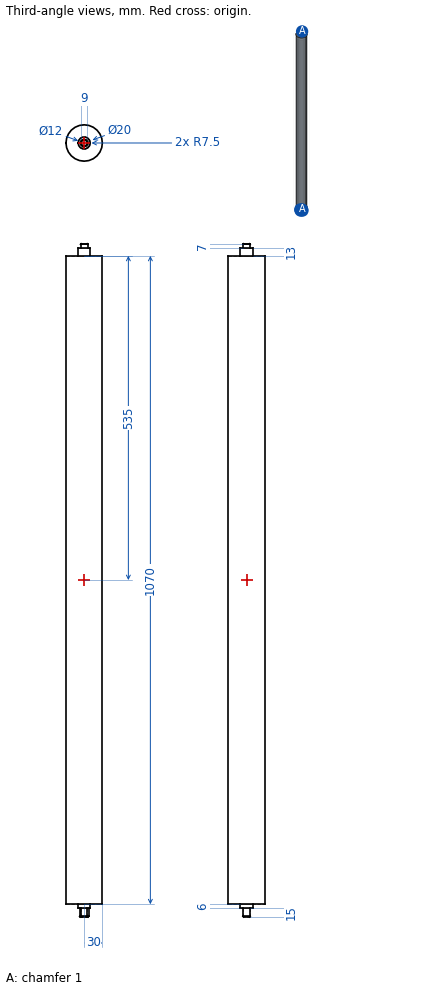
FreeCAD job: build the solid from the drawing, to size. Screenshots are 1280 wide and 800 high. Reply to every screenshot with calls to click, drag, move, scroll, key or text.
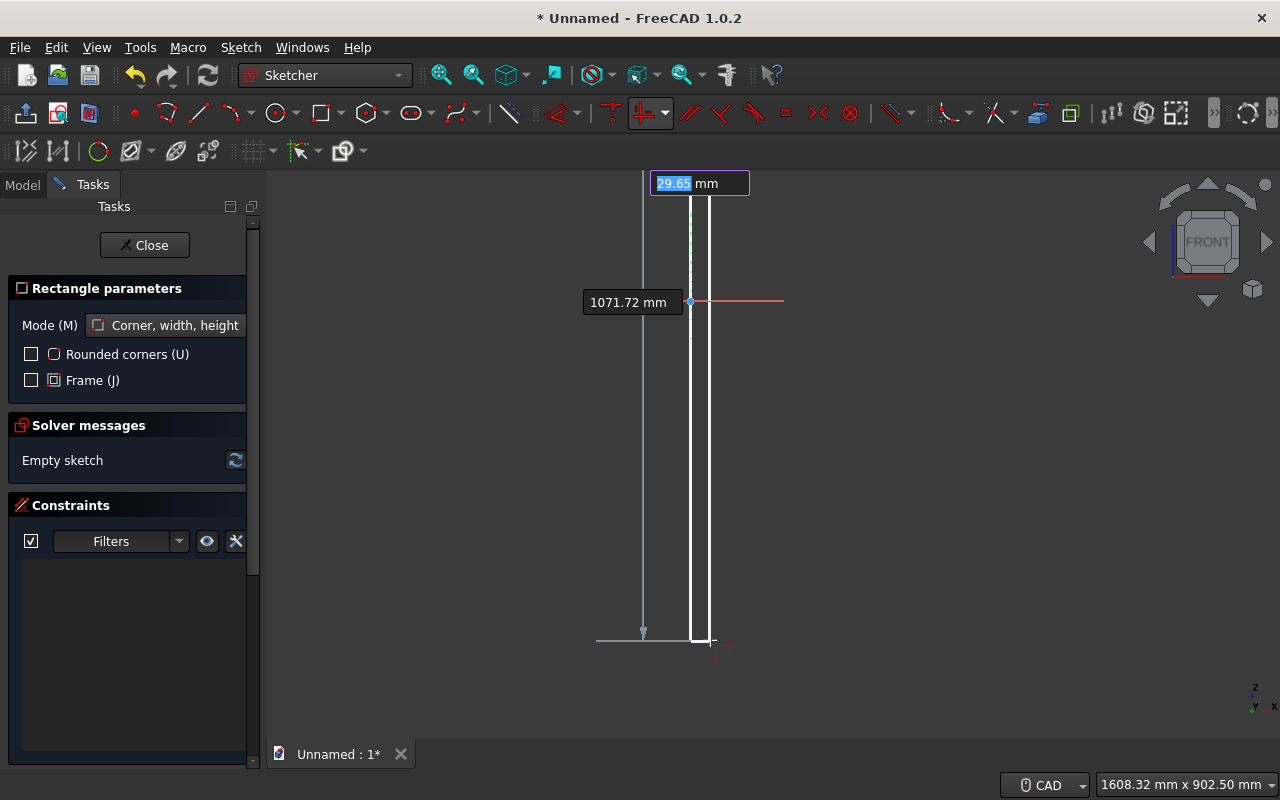
click(710, 639)
key(Escape)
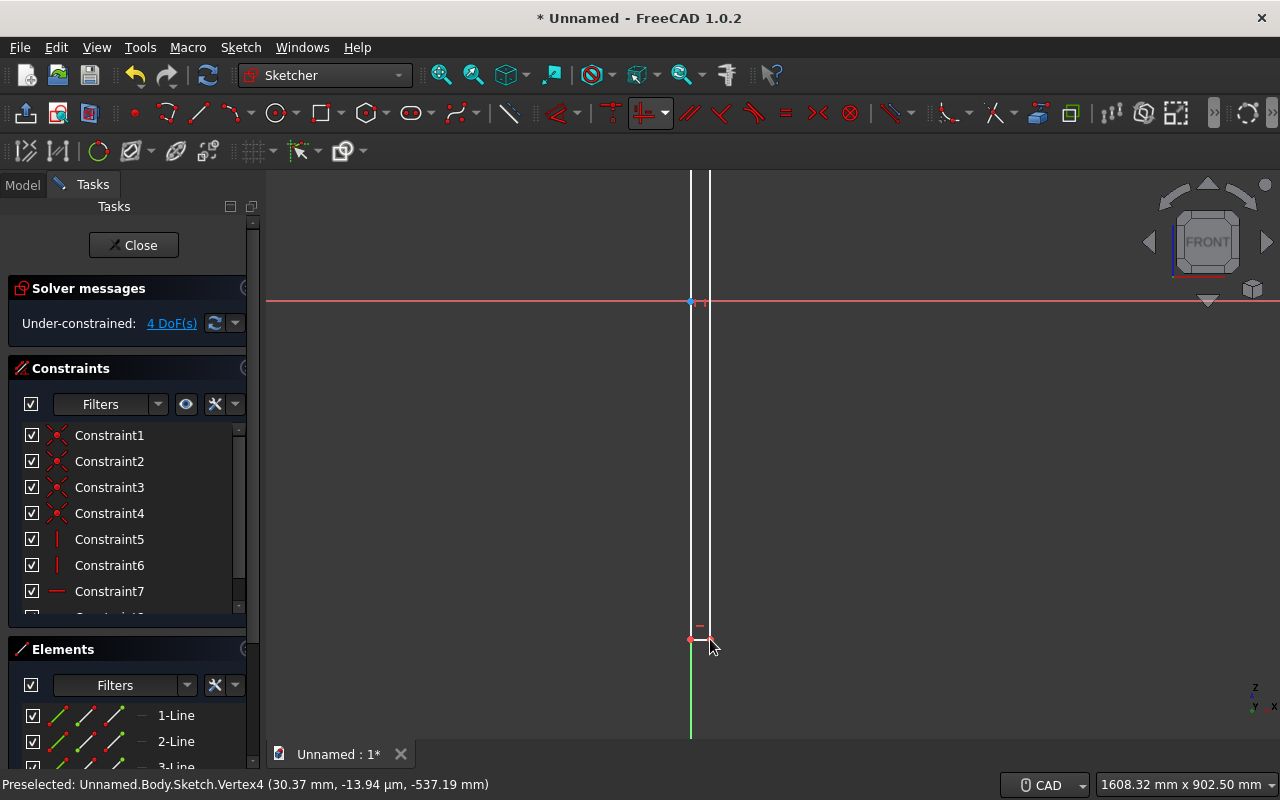
scroll(710, 641, down, 3)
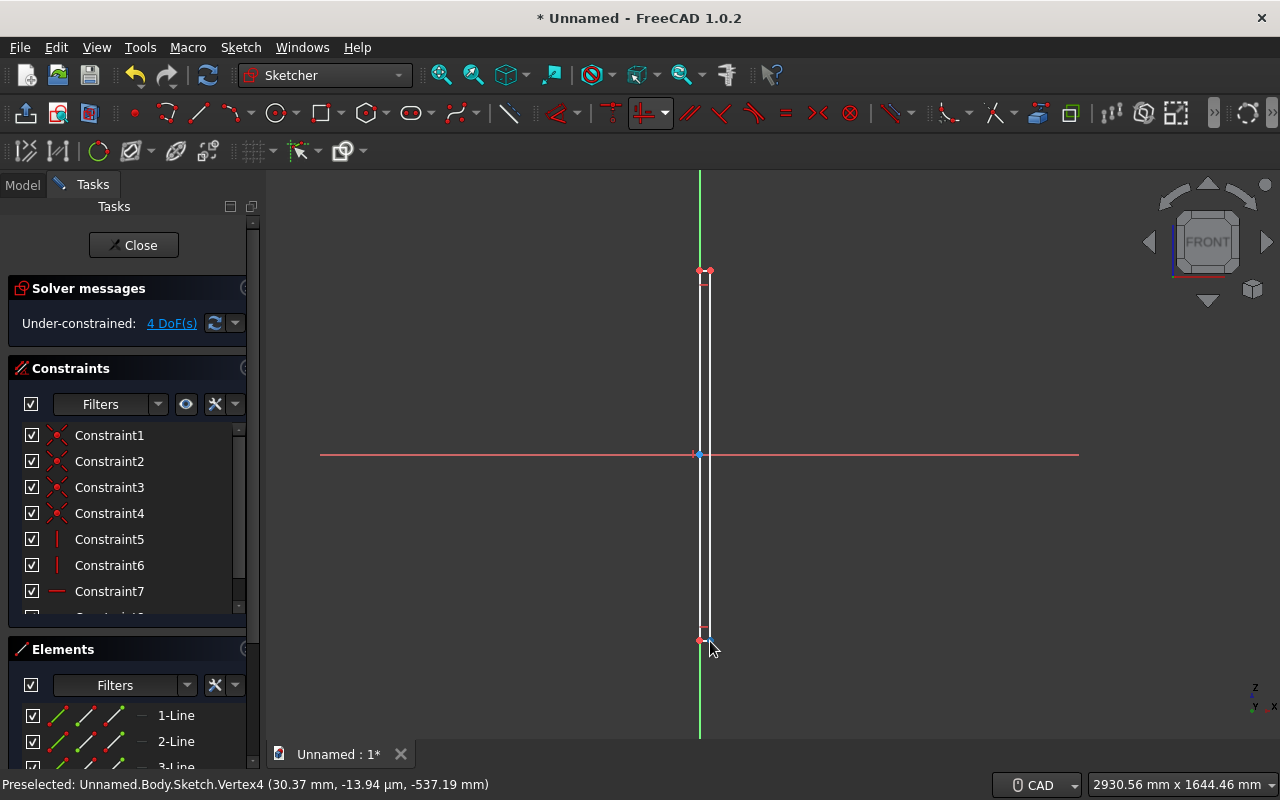
click(700, 271)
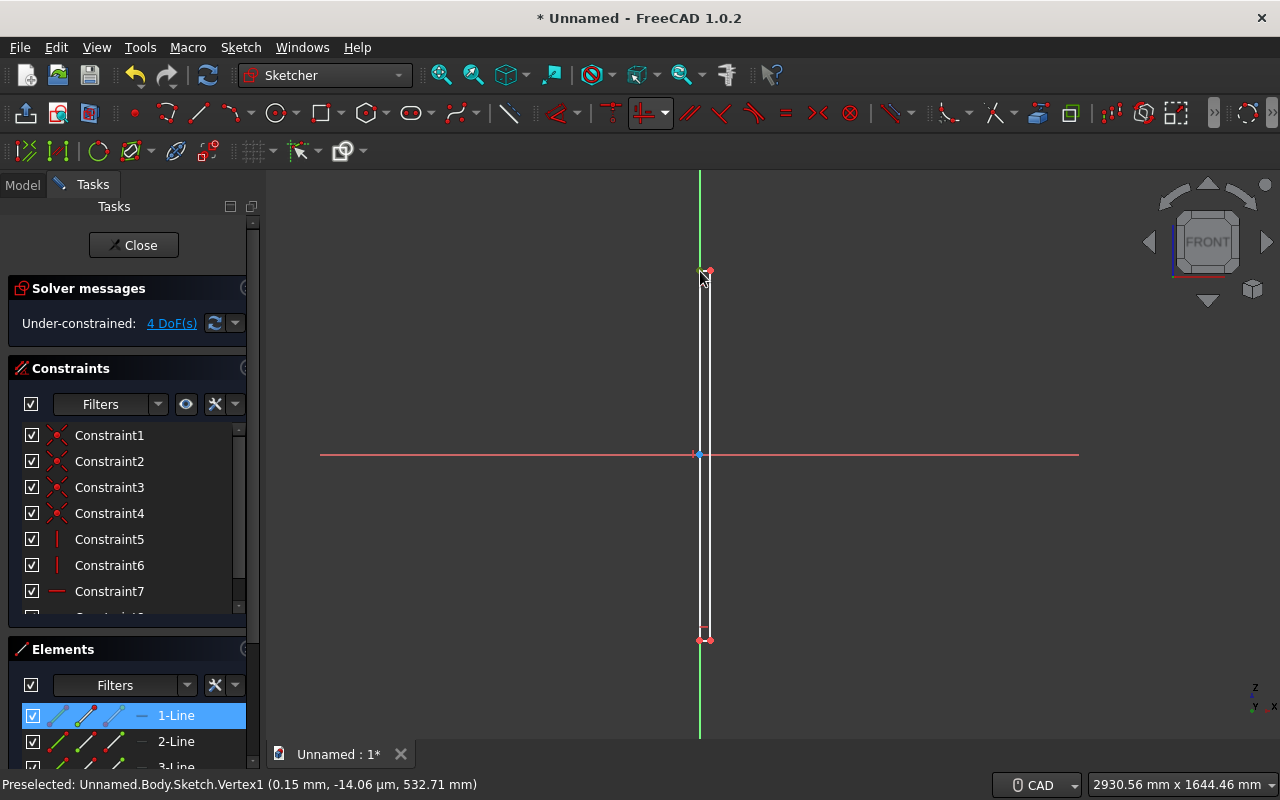
click(700, 674)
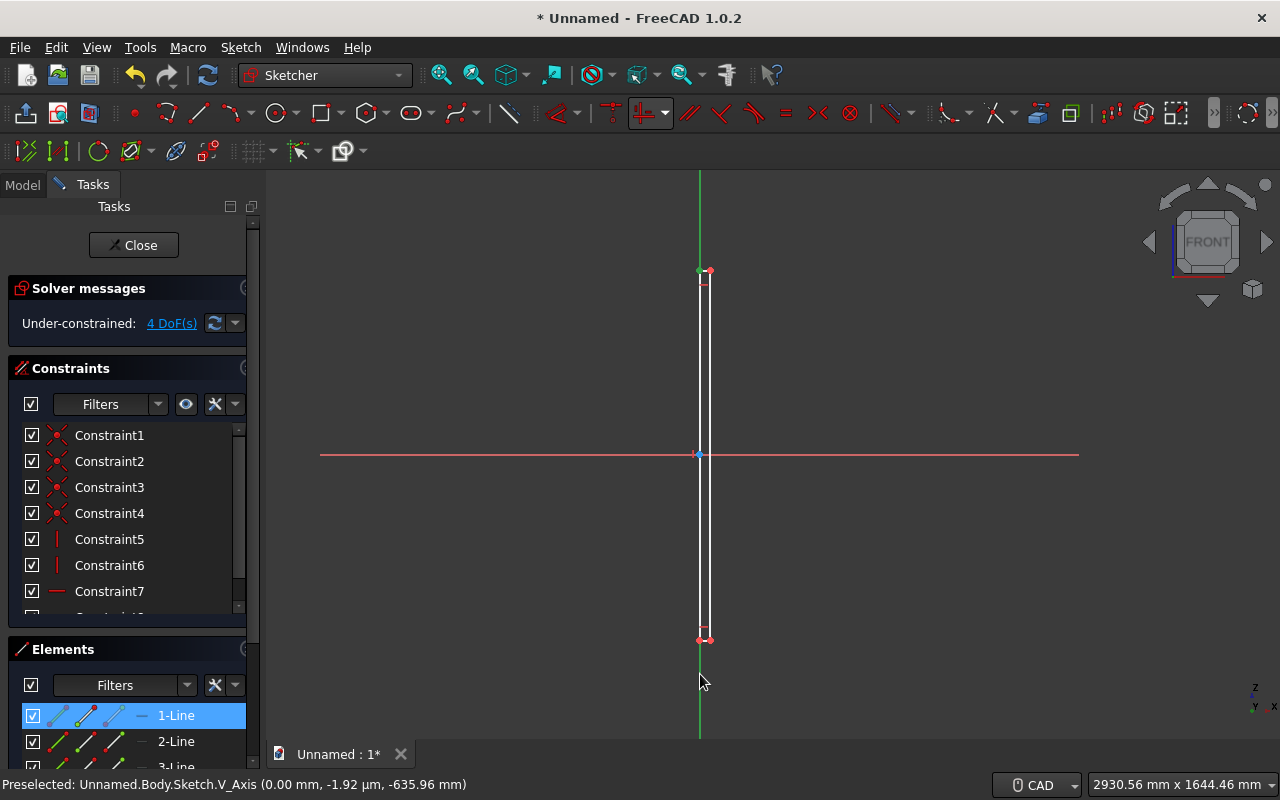
key(c)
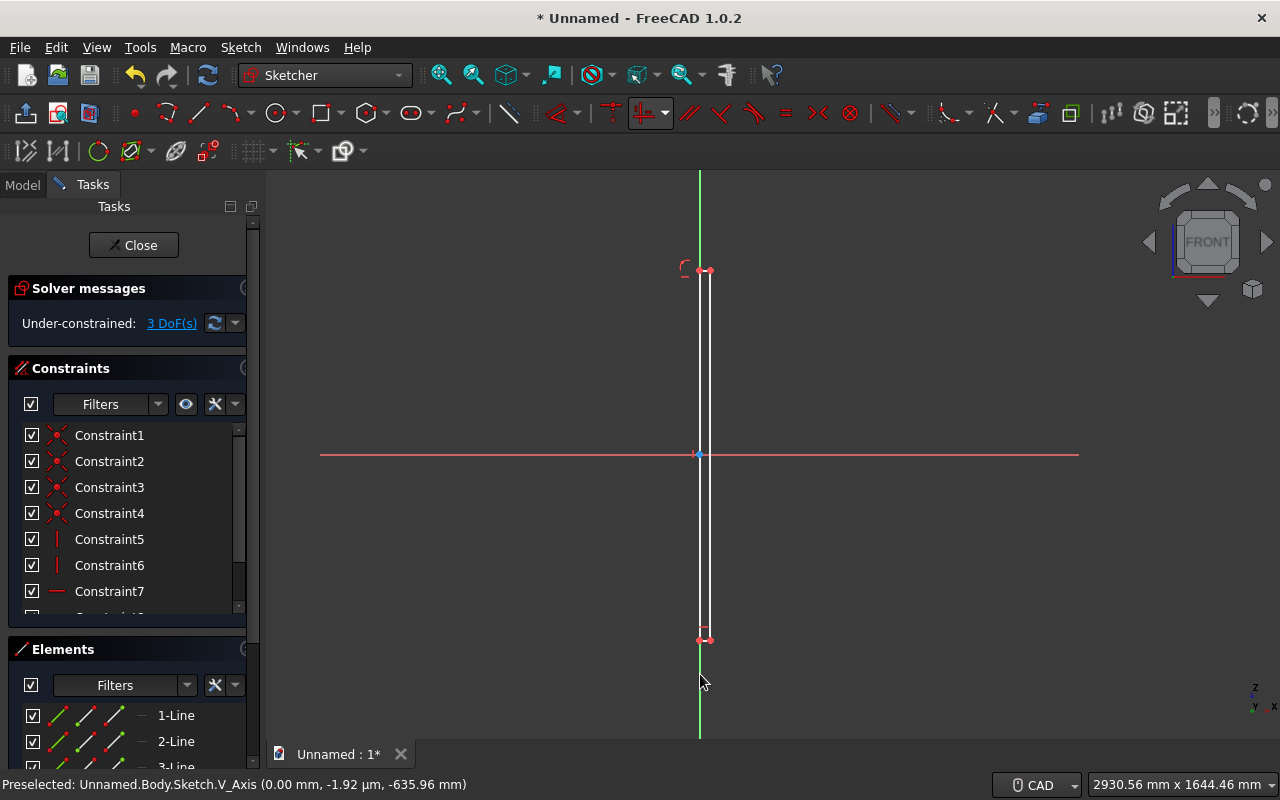
scroll(705, 641, up, 7)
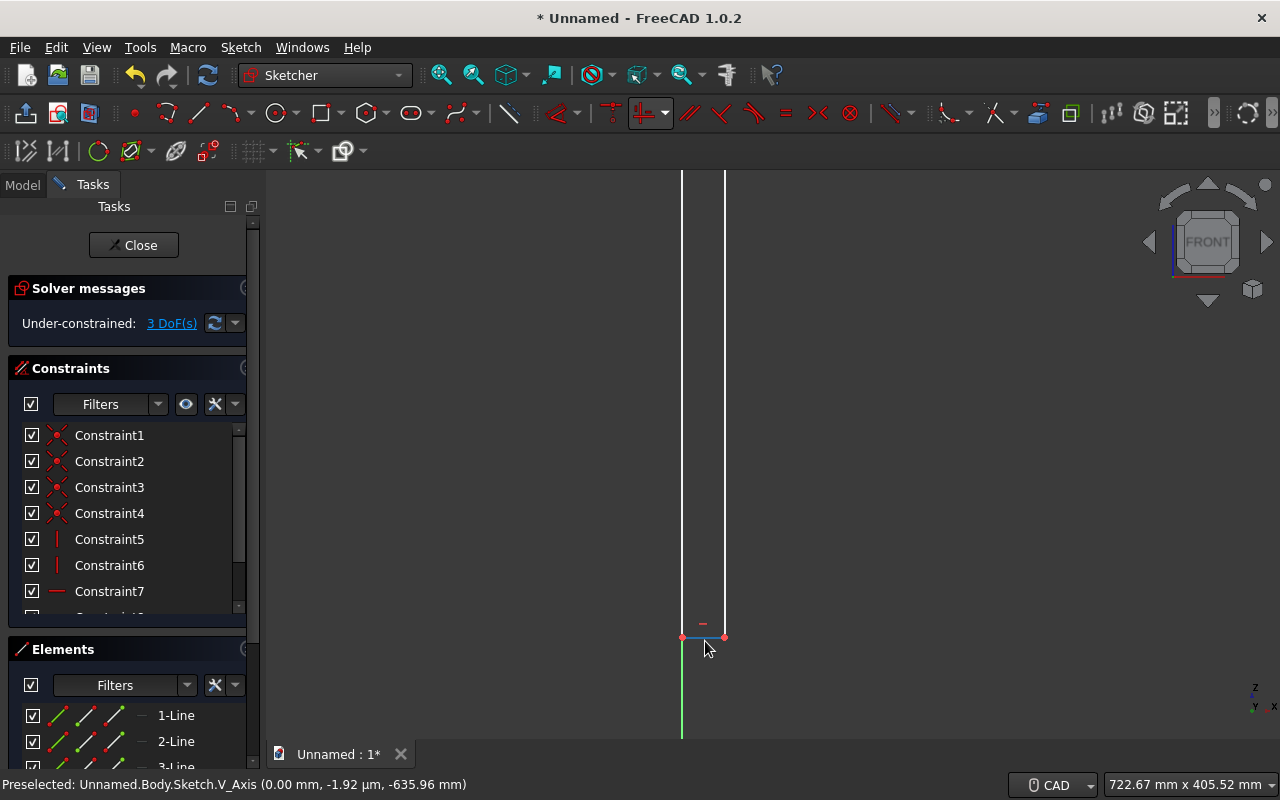
click(703, 638)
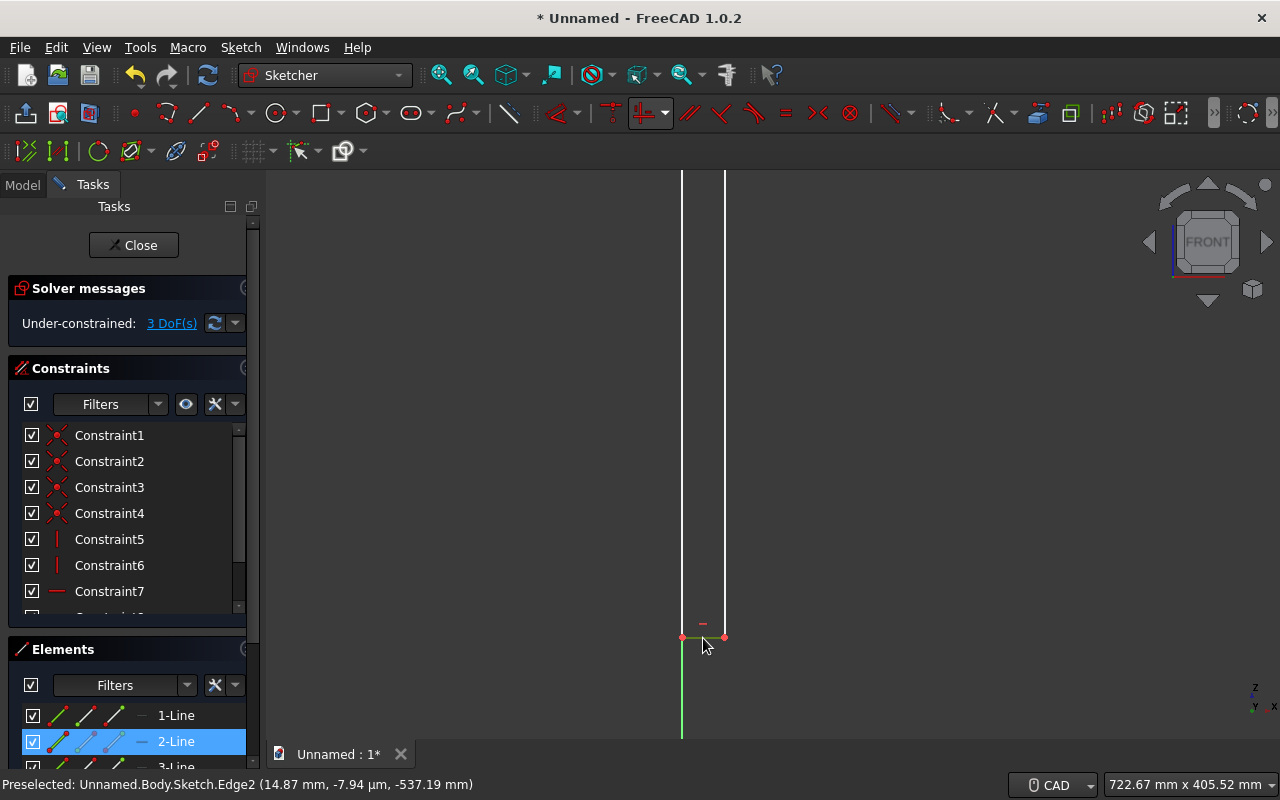
key(l)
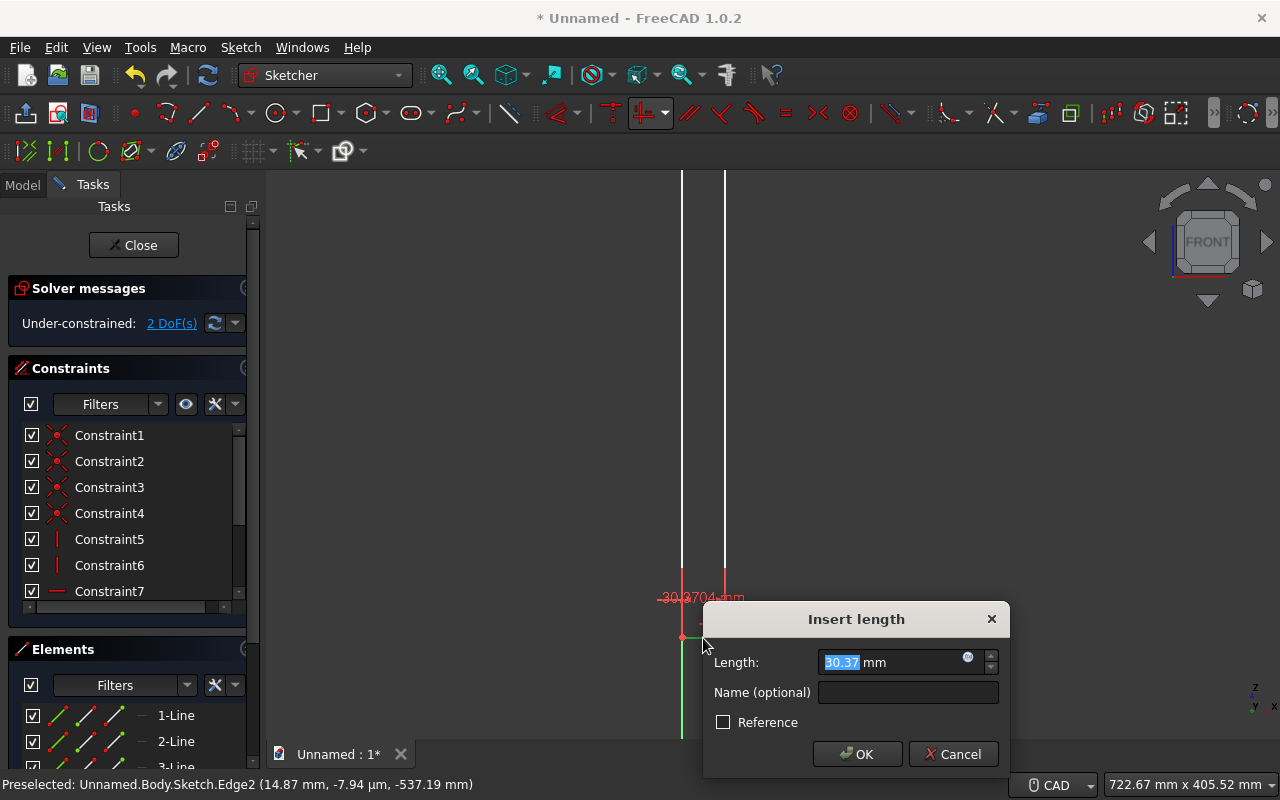
text(30)
key(Return)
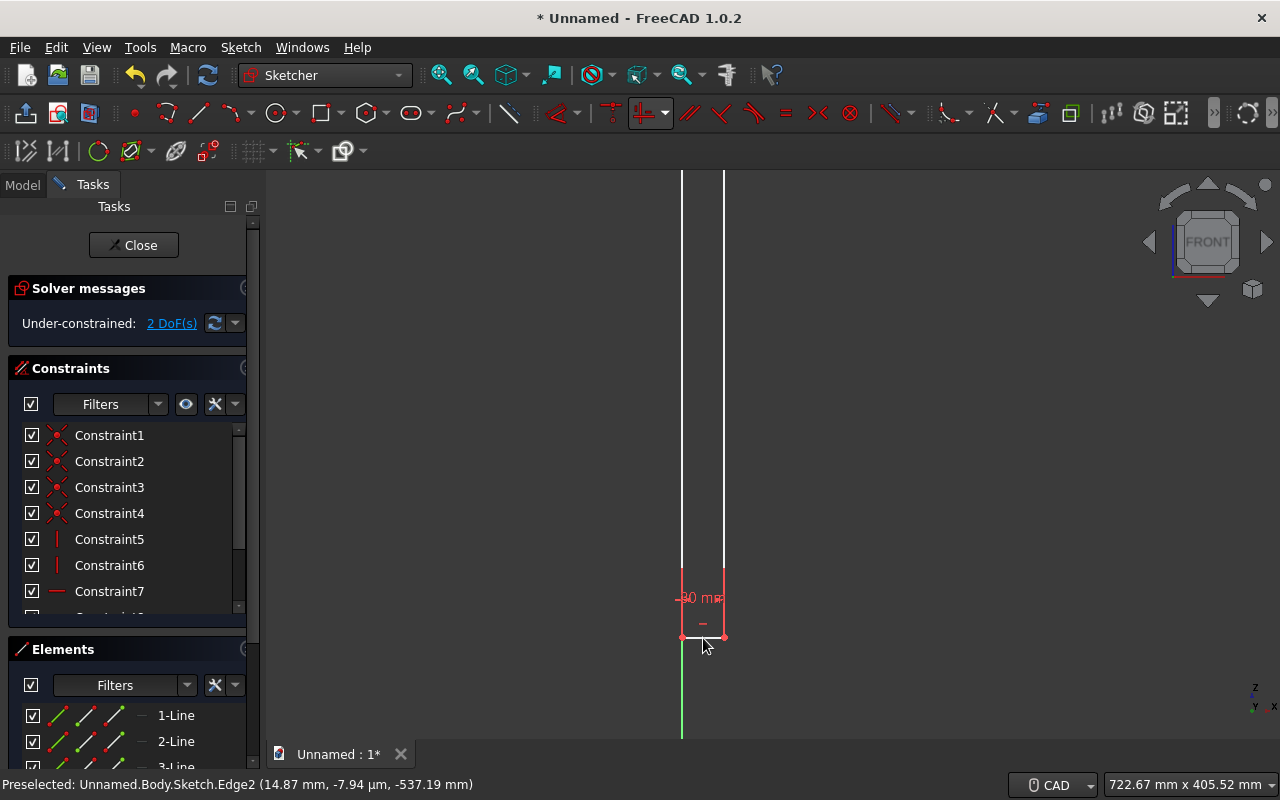
scroll(705, 641, down, 7)